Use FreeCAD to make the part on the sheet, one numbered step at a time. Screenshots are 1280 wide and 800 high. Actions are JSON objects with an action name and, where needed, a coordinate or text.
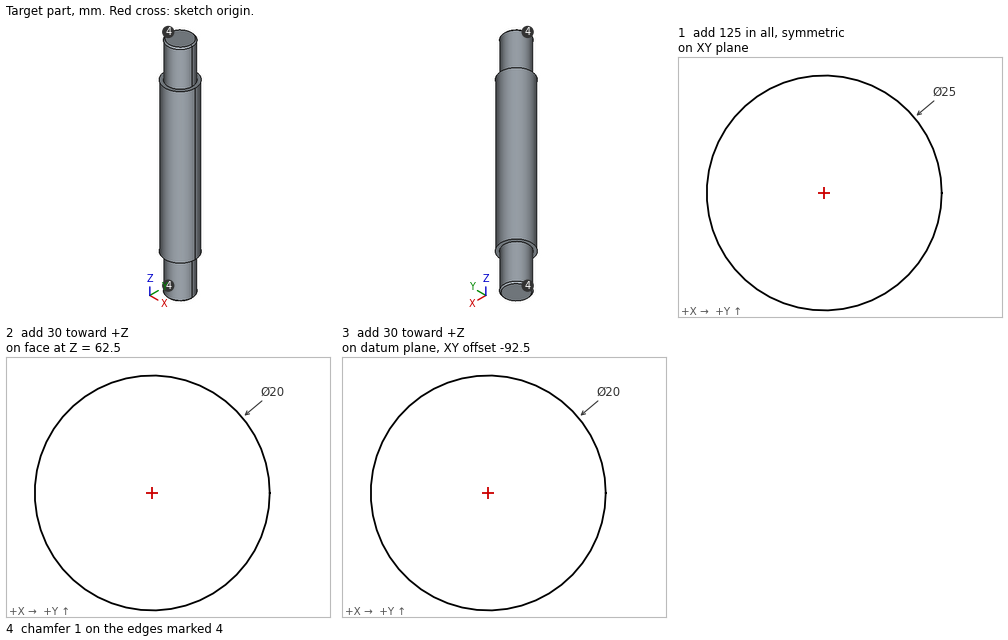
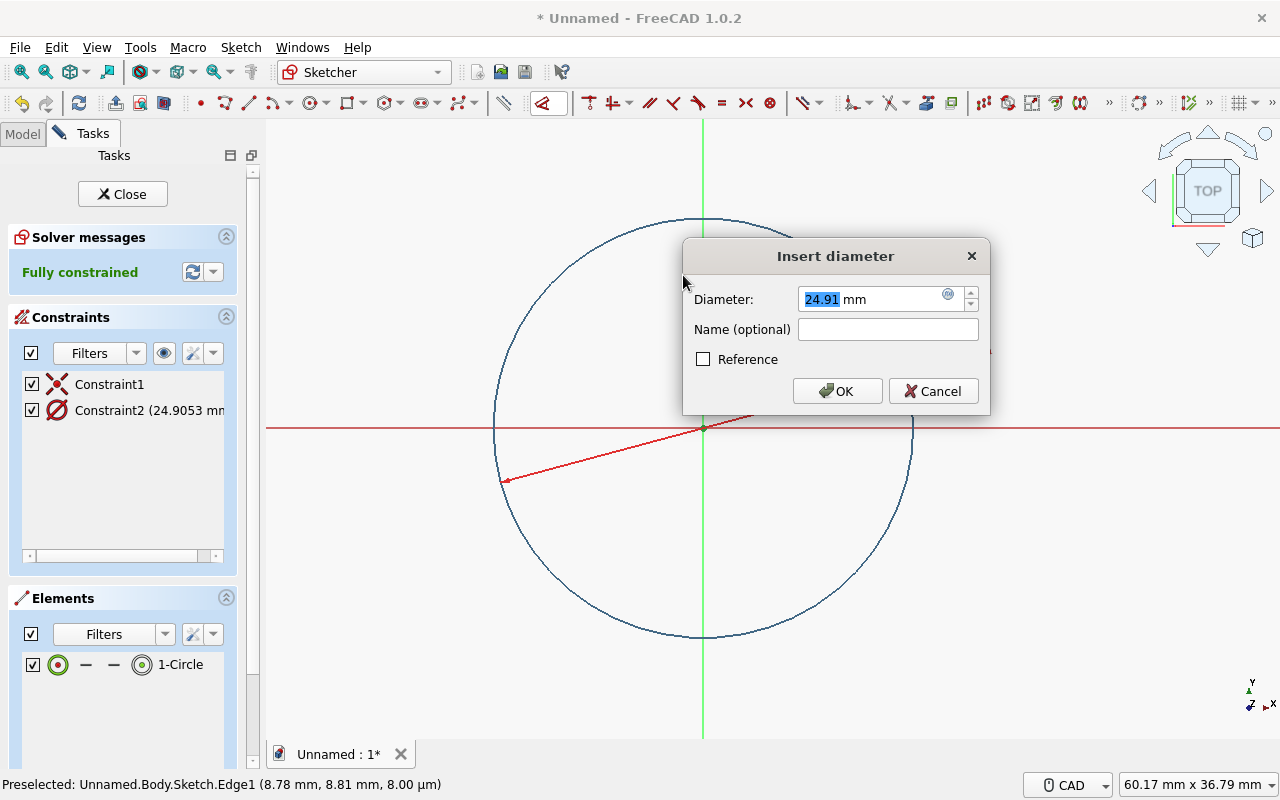
{"action": "type", "text": "25"}
{"action": "key", "text": "Return"}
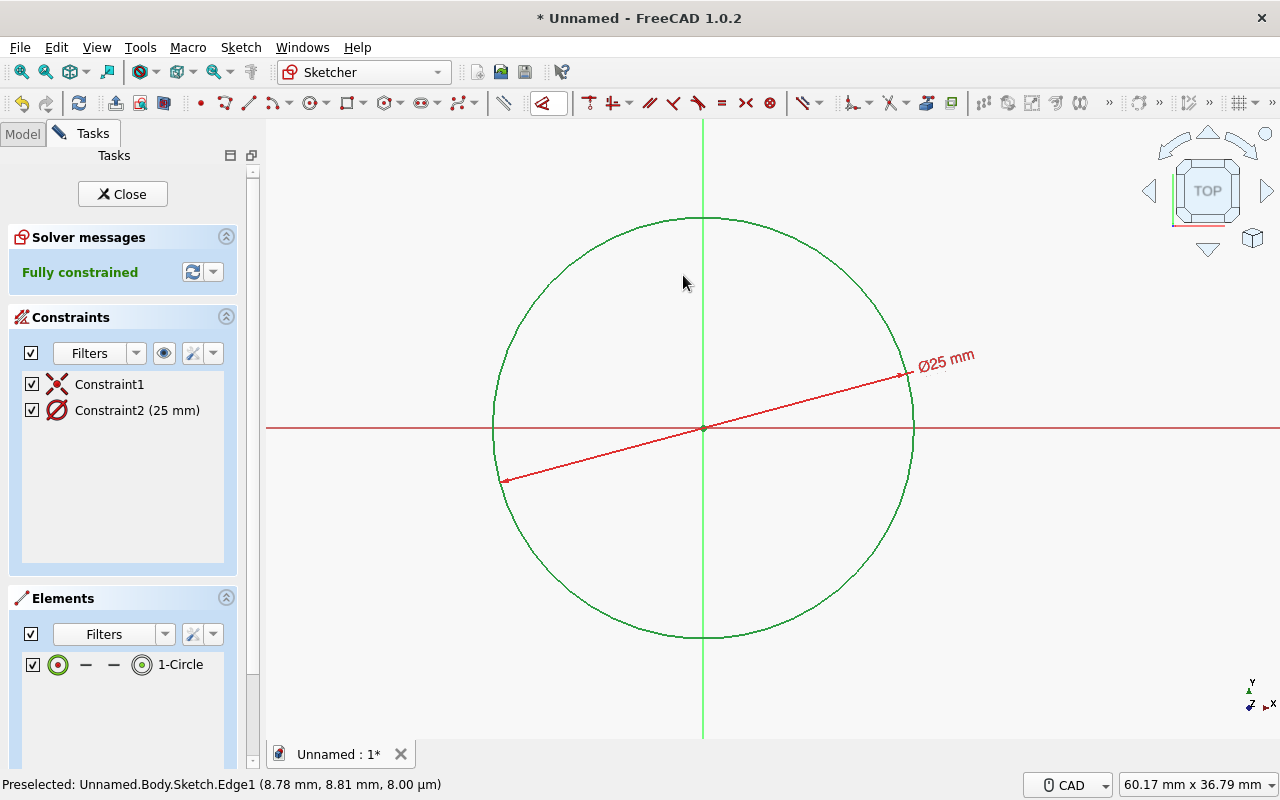
{"action": "left_click", "coordinate": [123, 194]}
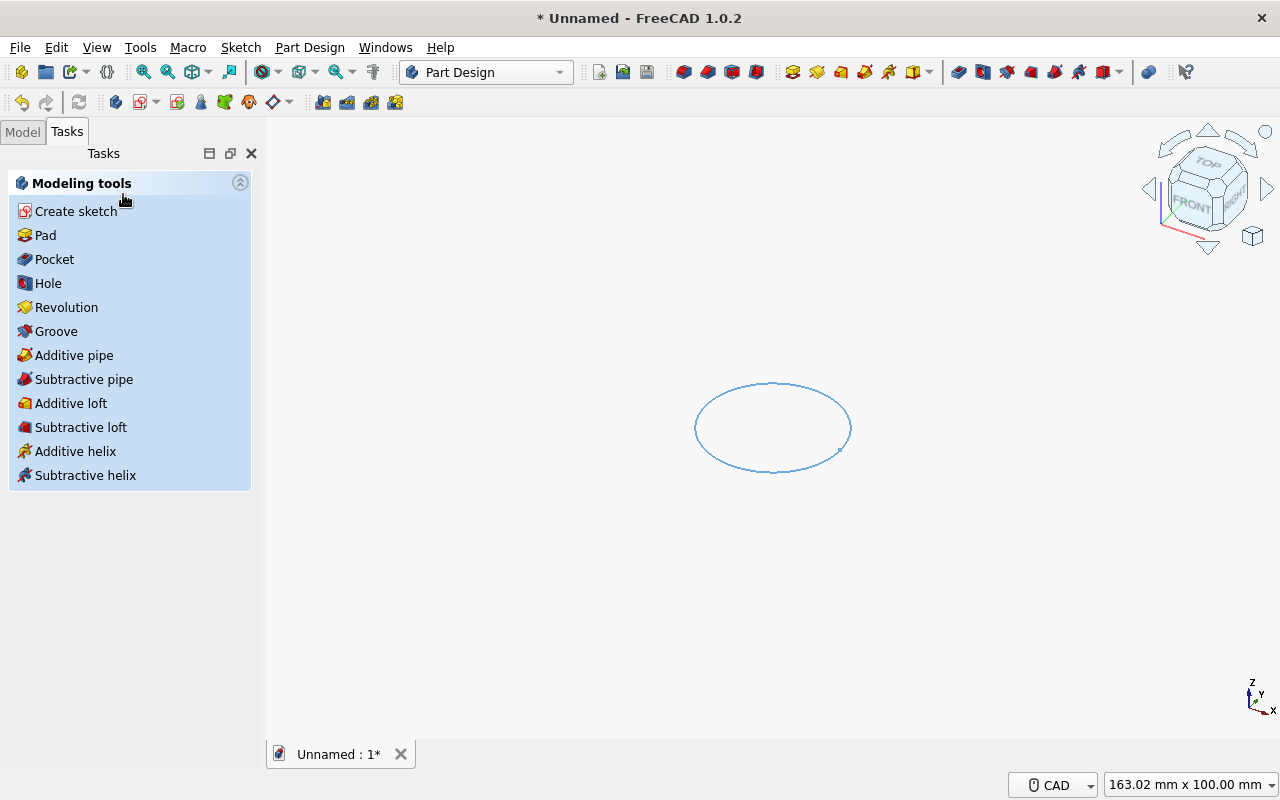
{"action": "left_click", "coordinate": [794, 72]}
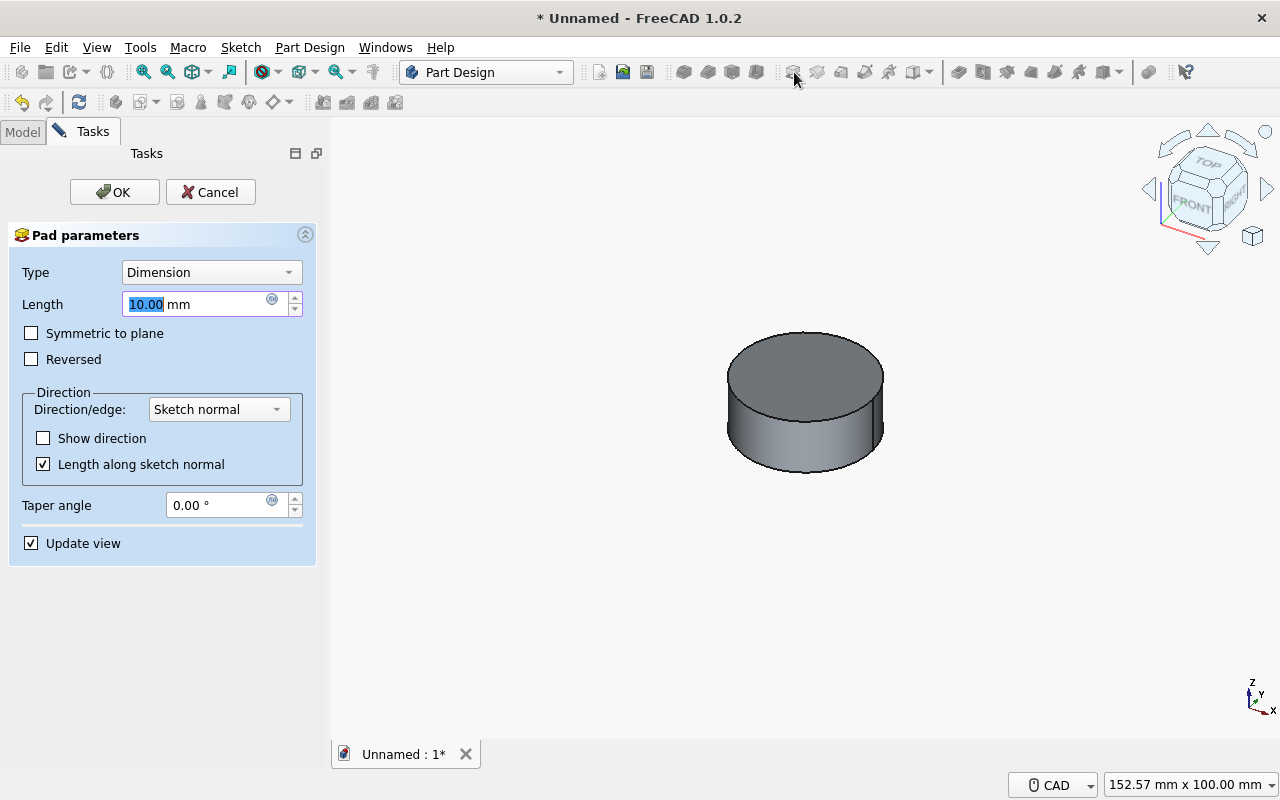
{"action": "type", "text": "125"}
{"action": "key", "text": "Tab"}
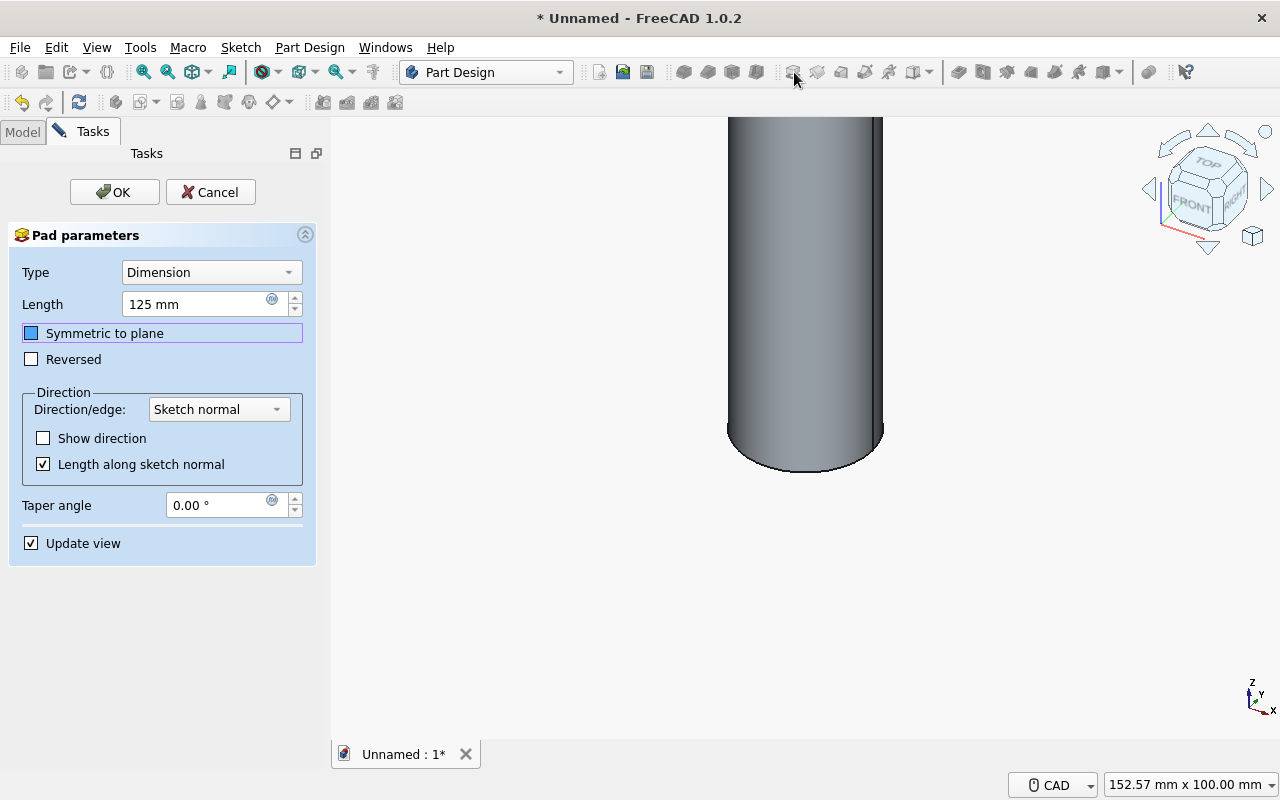
{"action": "left_click", "coordinate": [30, 333]}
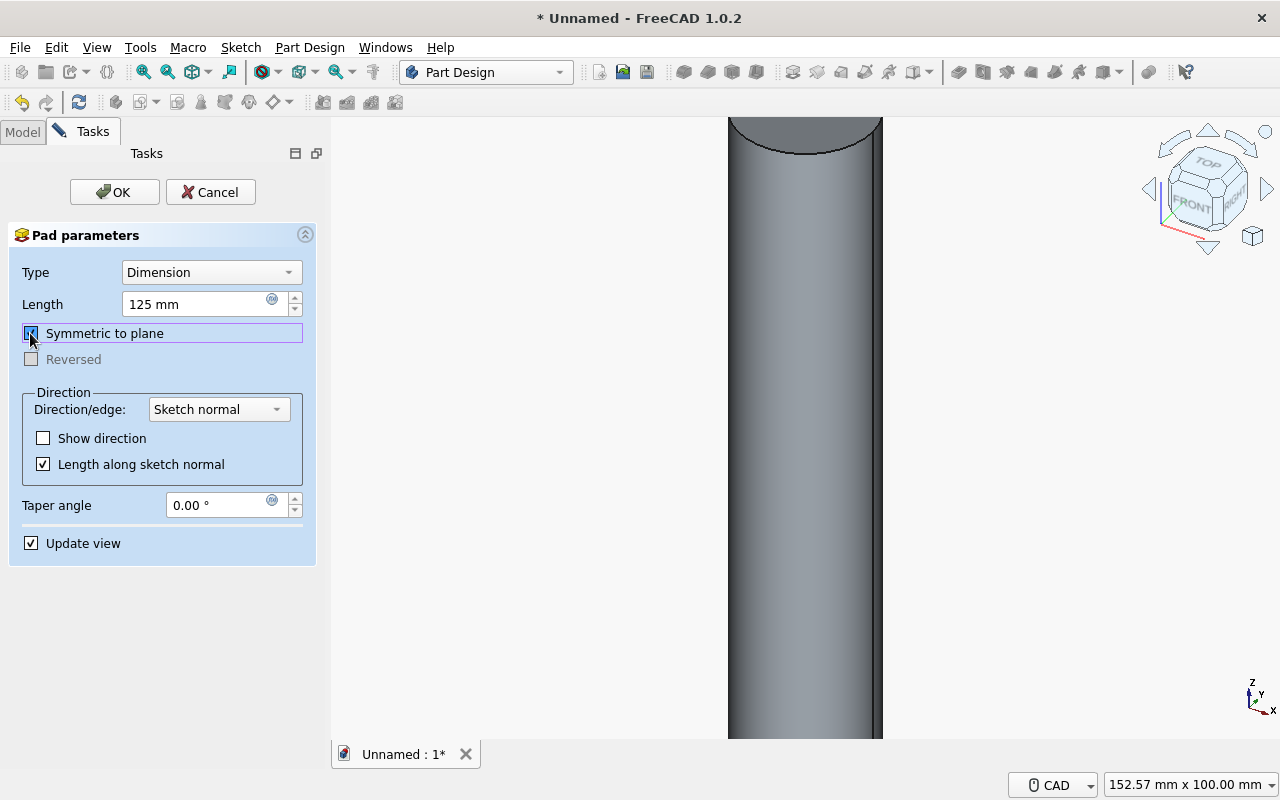
{"action": "left_click", "coordinate": [115, 192]}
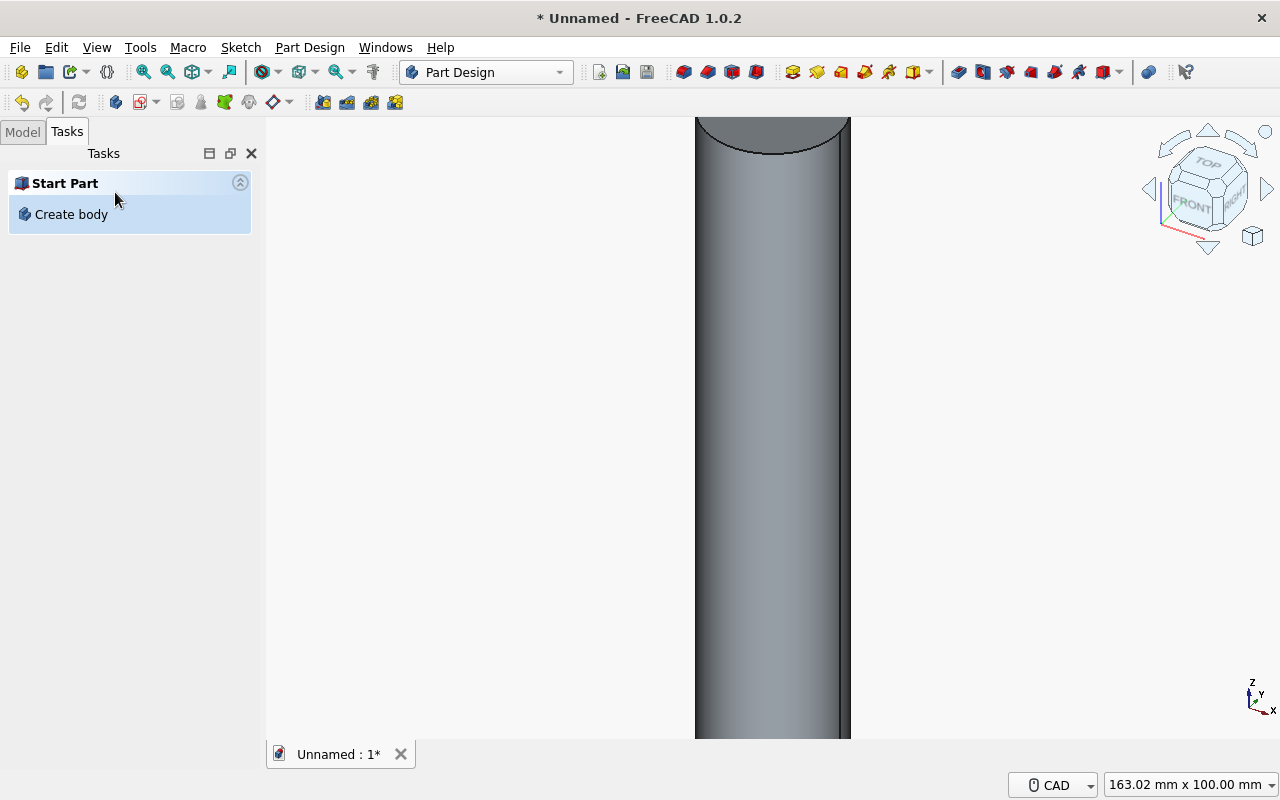
{"action": "left_click", "coordinate": [144, 72]}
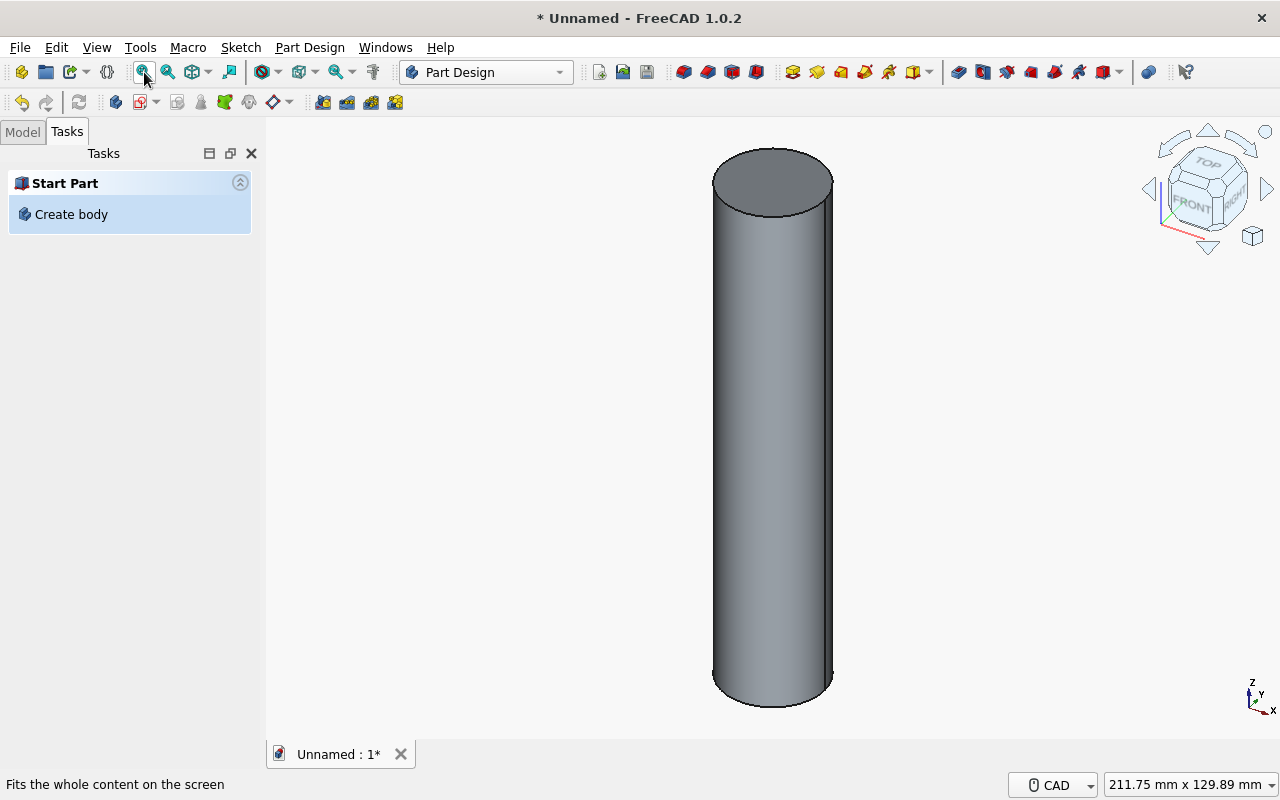
{"action": "left_click", "coordinate": [773, 182]}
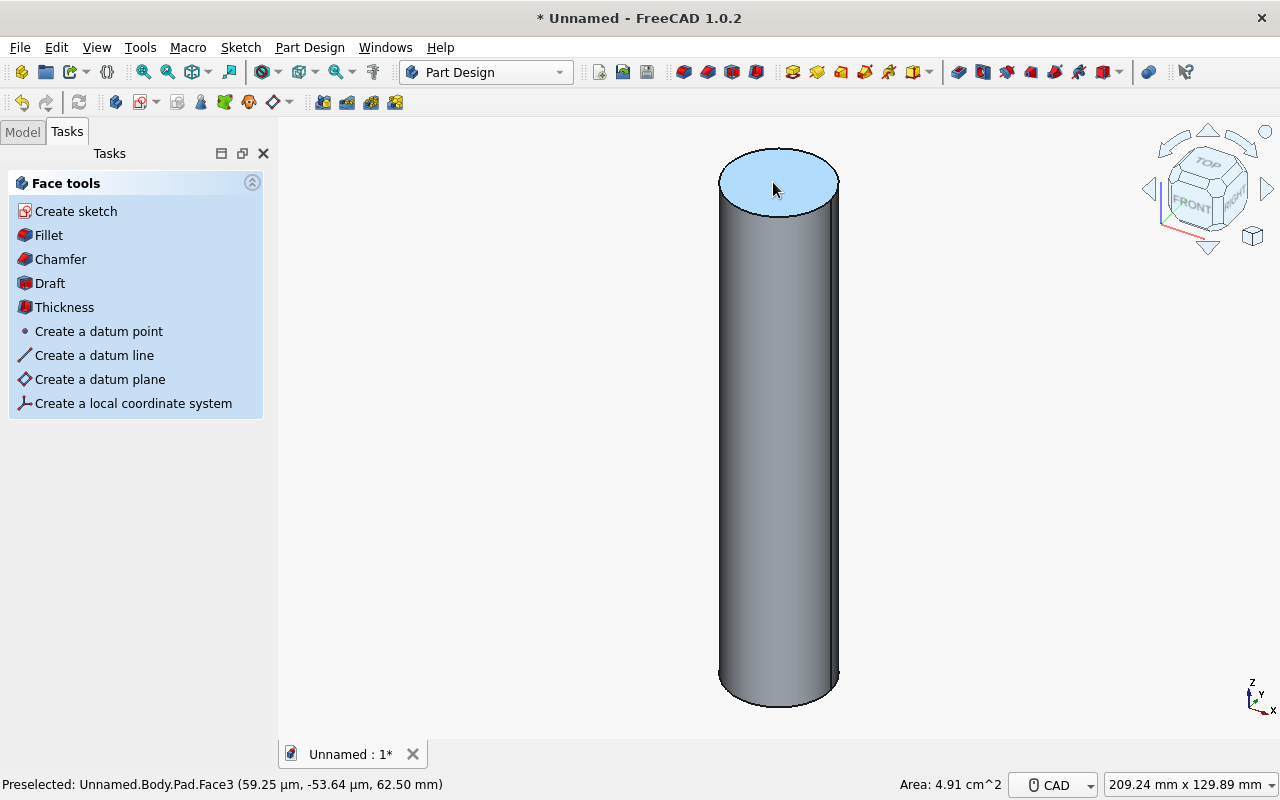
{"action": "left_click", "coordinate": [140, 102]}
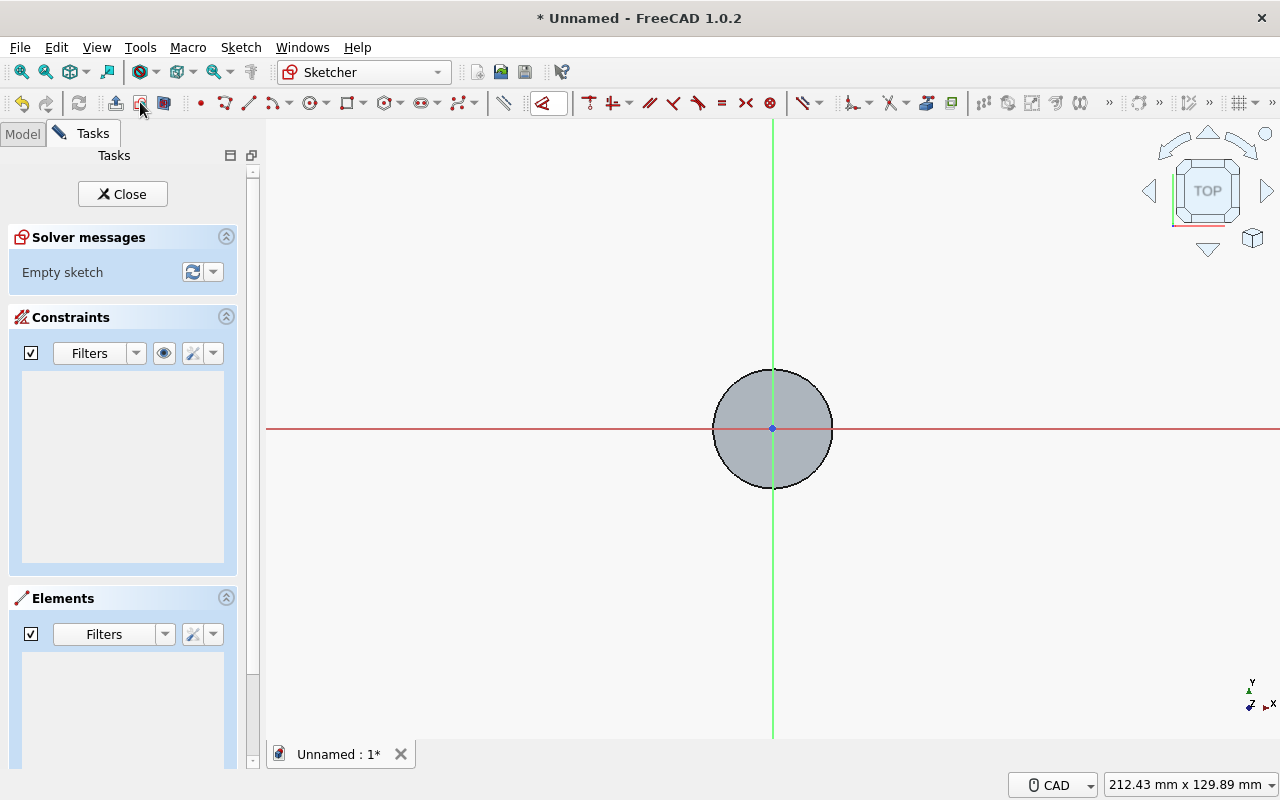
{"action": "scroll", "coordinate": [795, 429], "scroll_direction": "up", "scroll_amount": 7}